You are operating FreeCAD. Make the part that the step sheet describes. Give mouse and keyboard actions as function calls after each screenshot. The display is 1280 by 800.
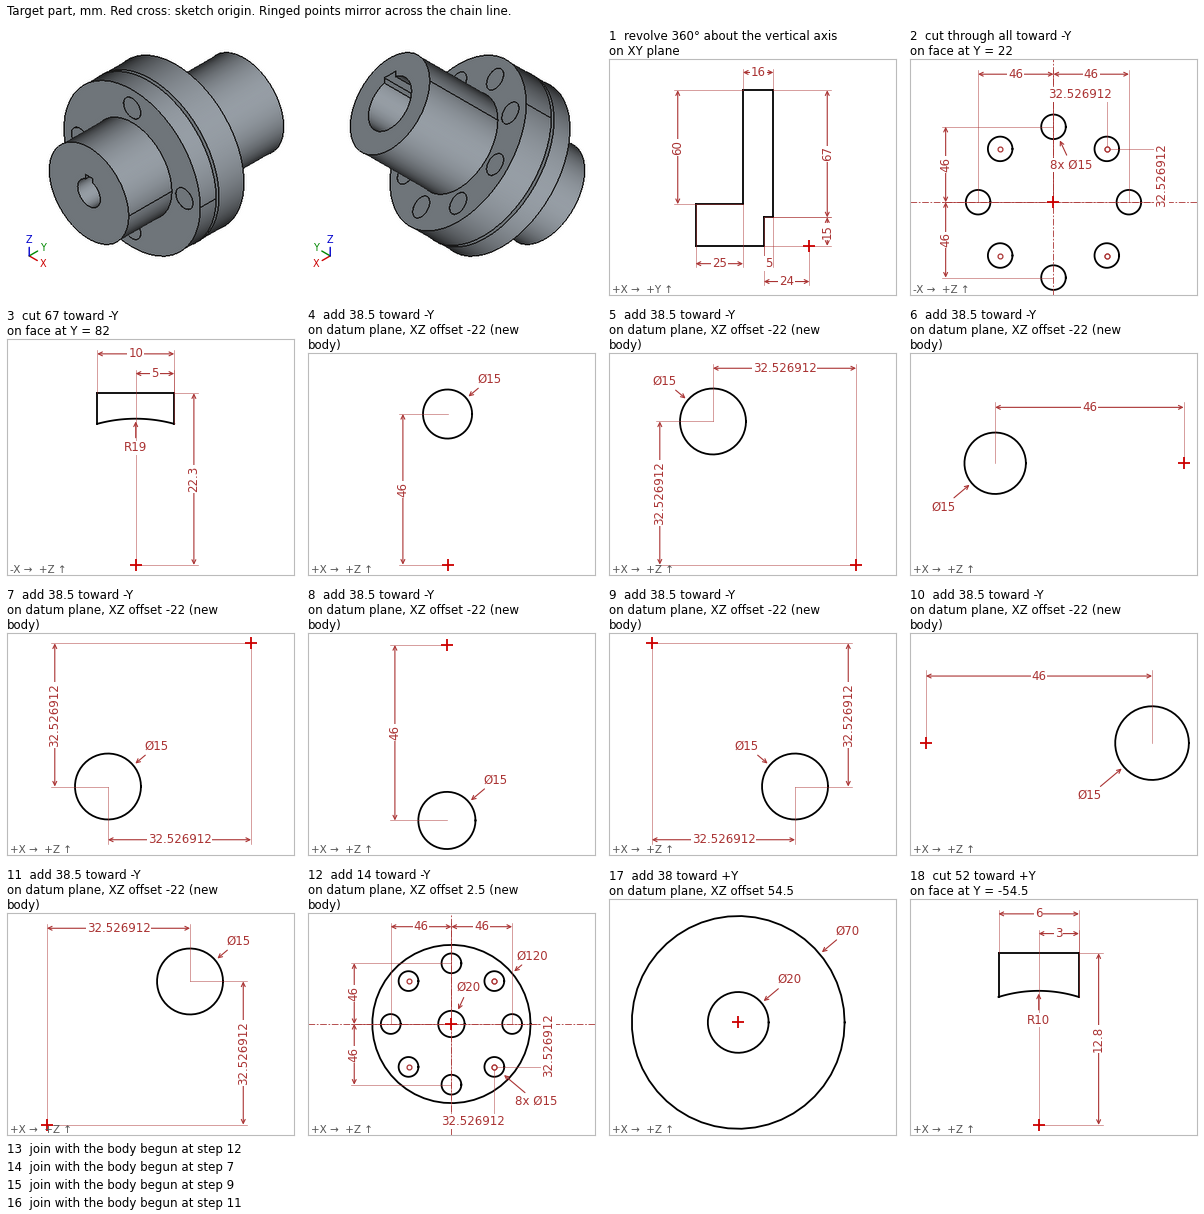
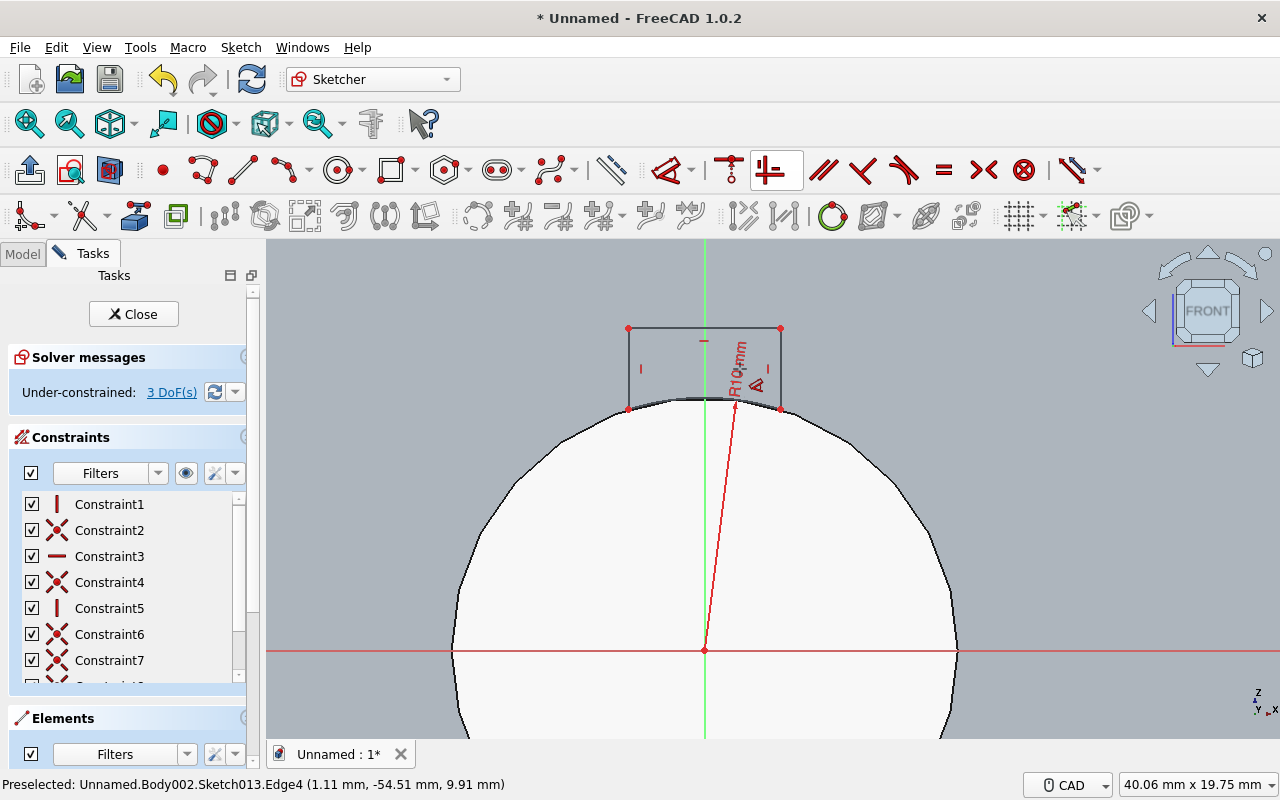
click(735, 328)
click(670, 294)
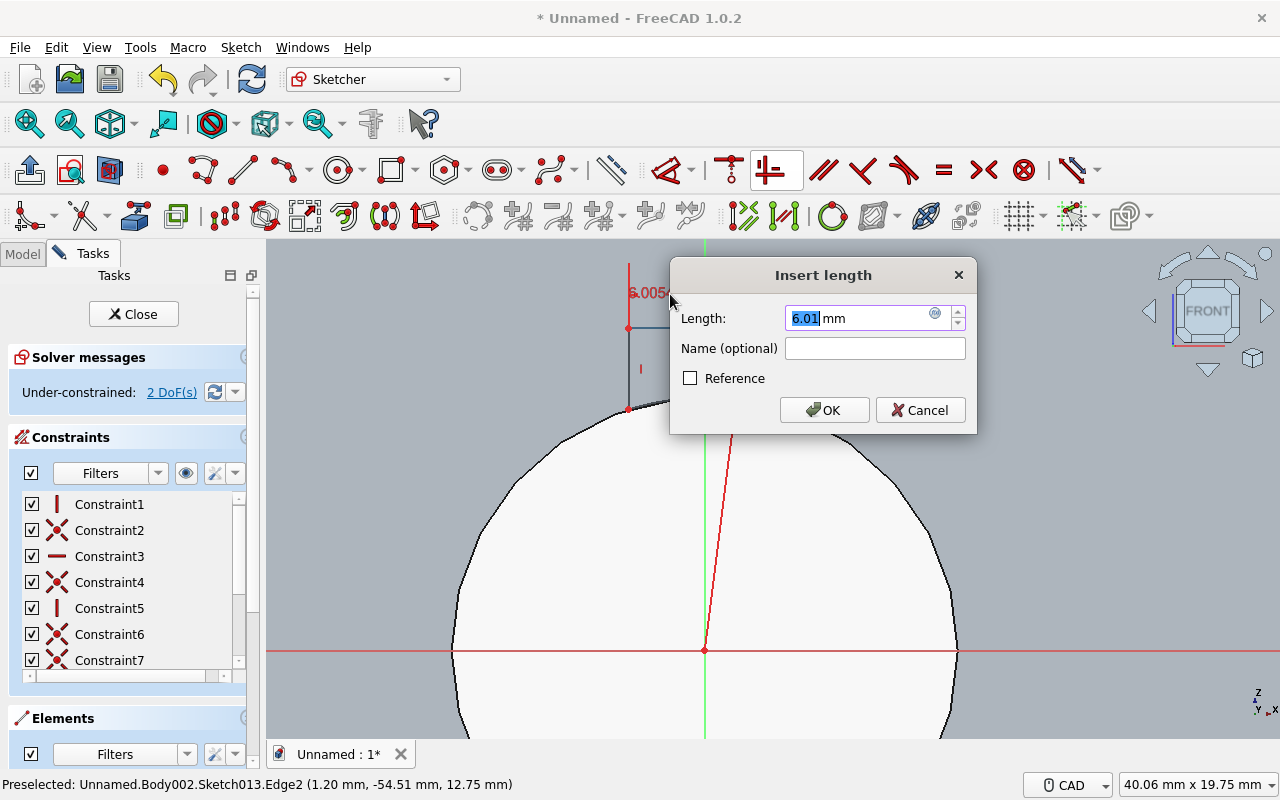
text(6)
key(Return)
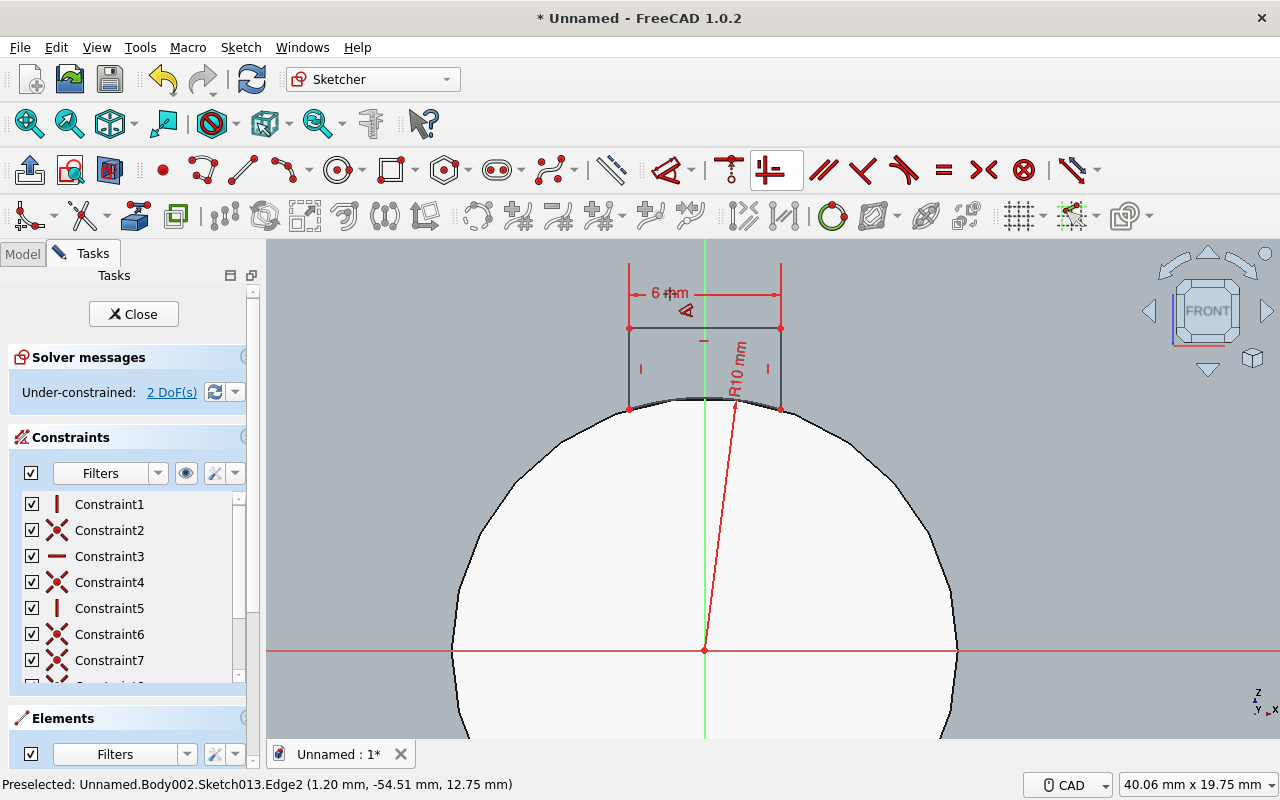
click(781, 410)
click(743, 685)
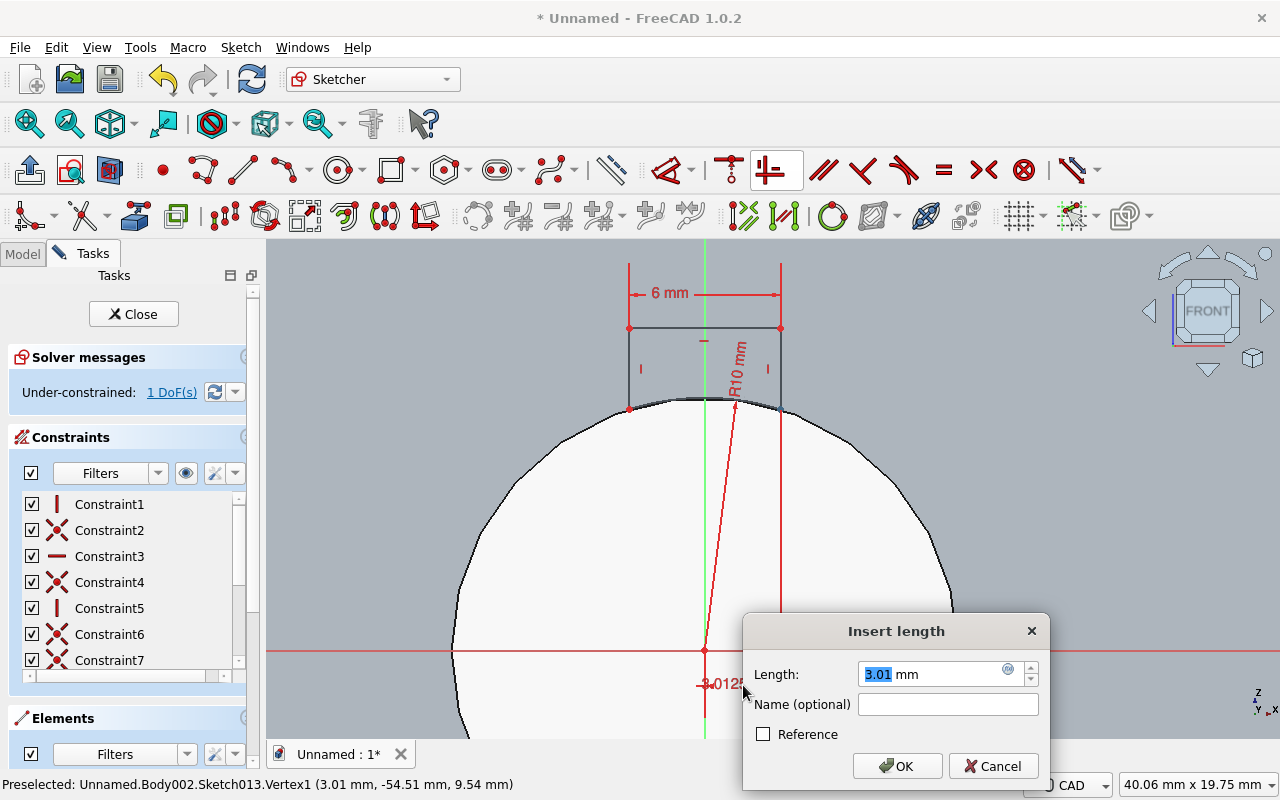
text(3)
key(Return)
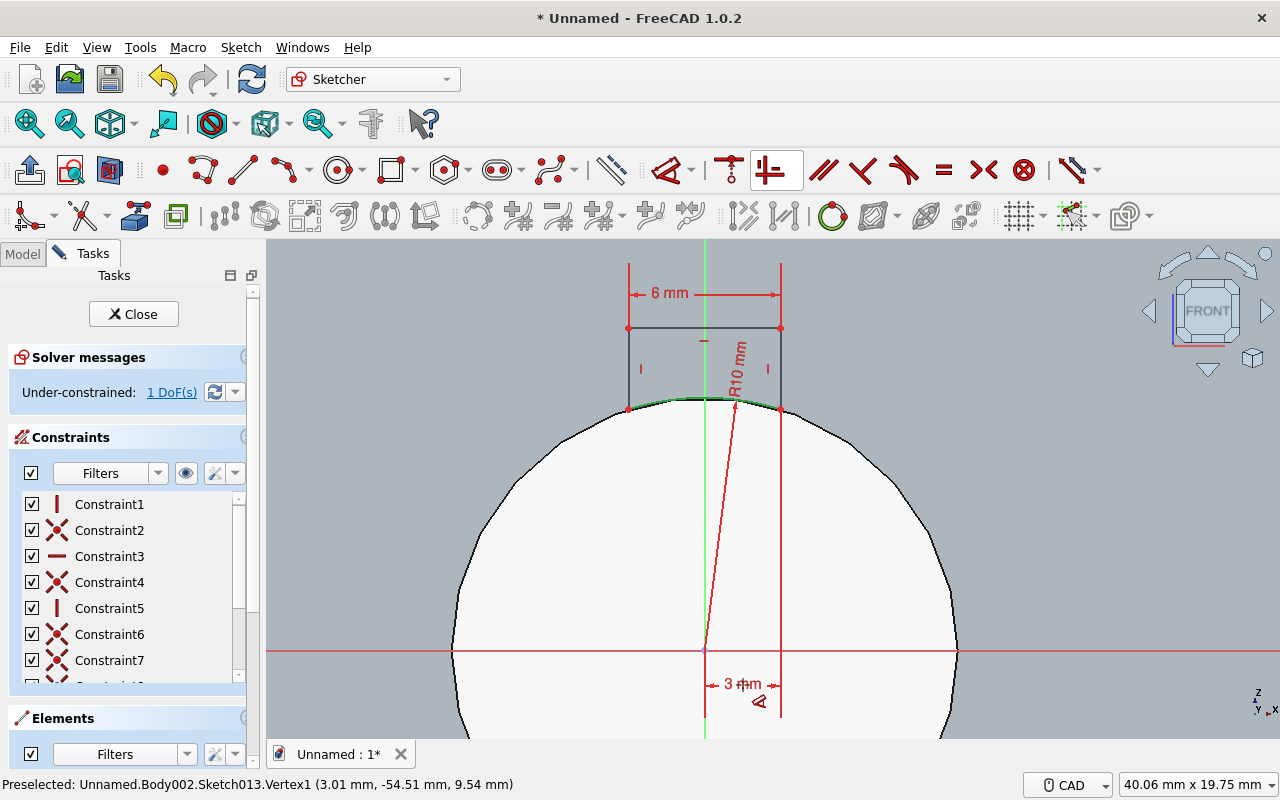
click(781, 328)
click(815, 490)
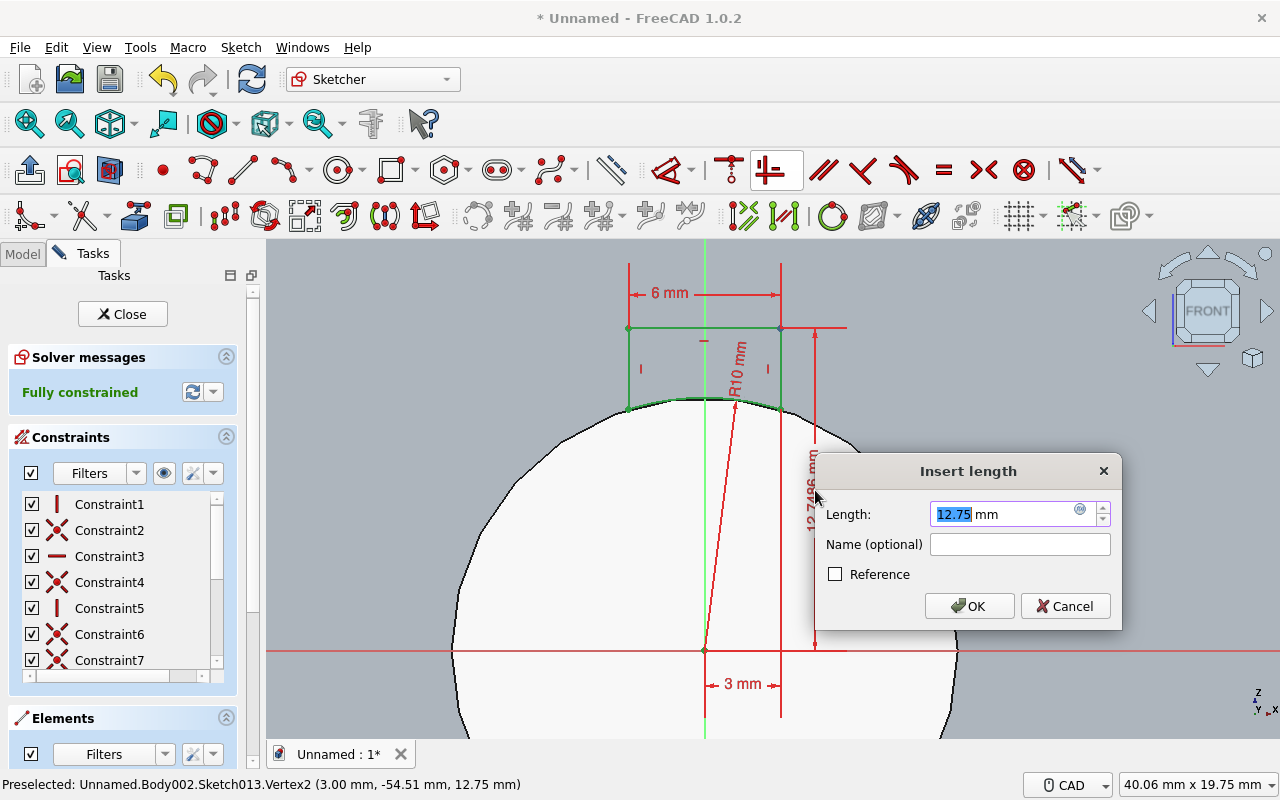
text(12.8)
key(Return)
key(Escape)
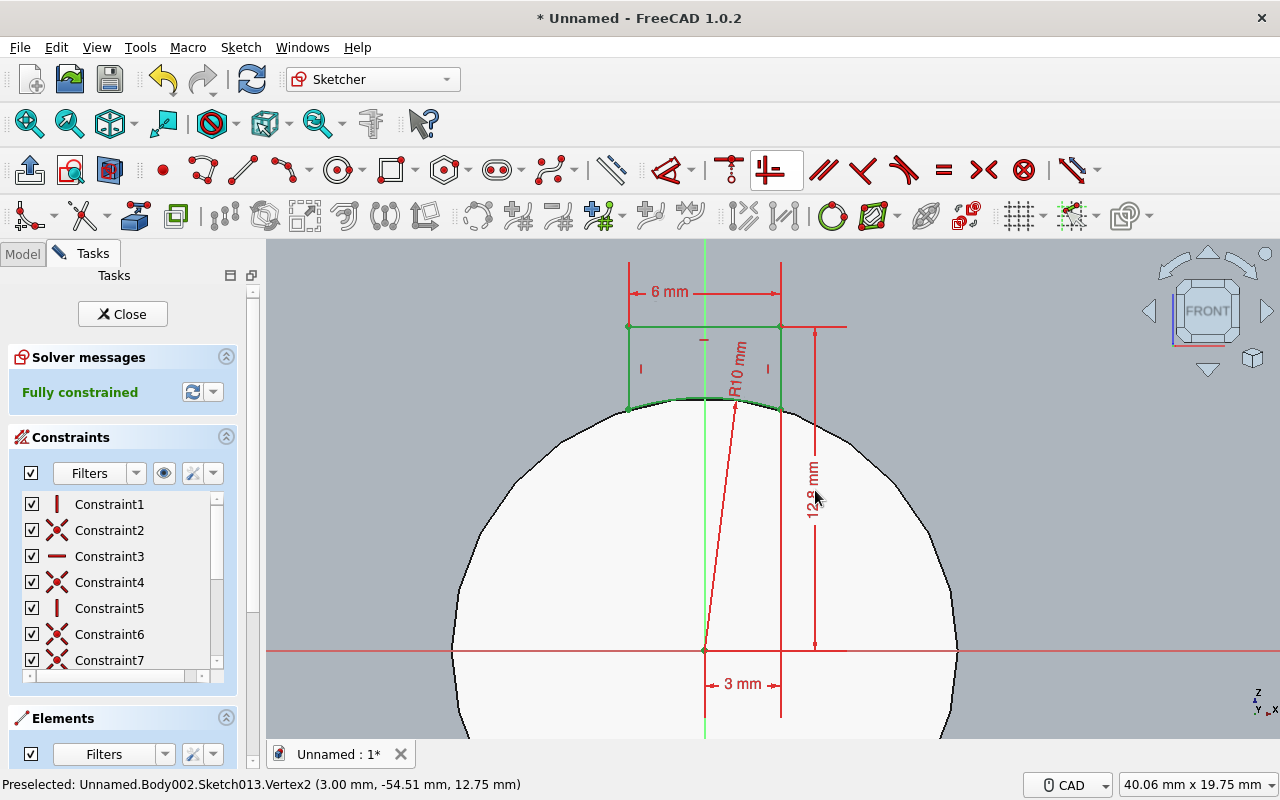
click(123, 314)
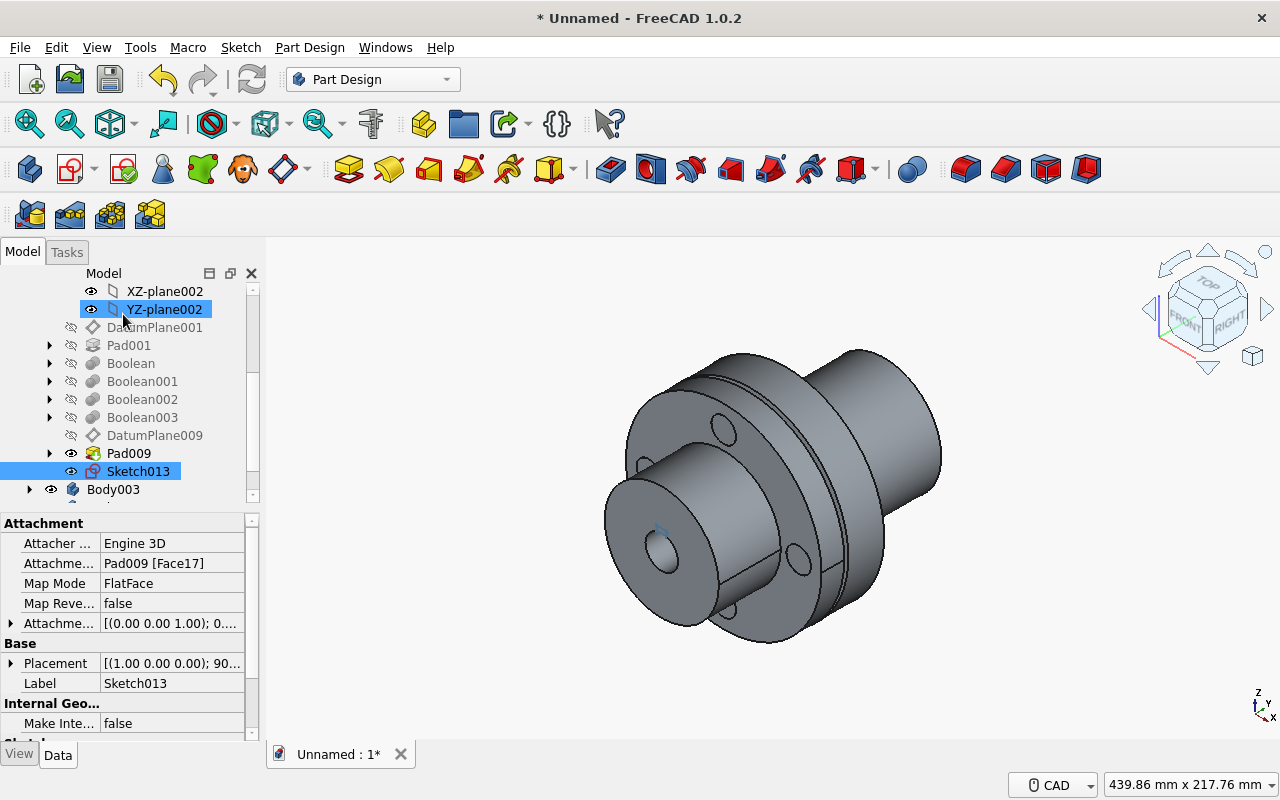
click(612, 170)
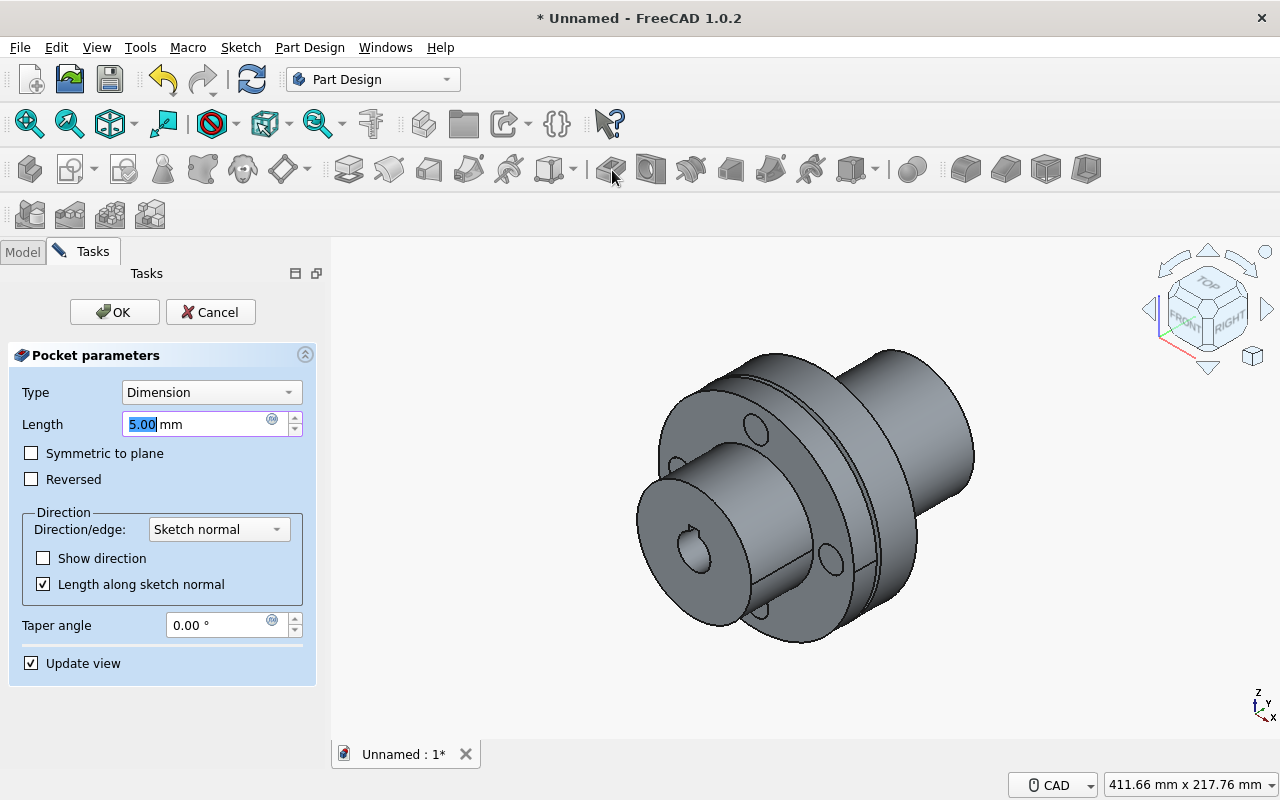
text(52)
key(Tab)